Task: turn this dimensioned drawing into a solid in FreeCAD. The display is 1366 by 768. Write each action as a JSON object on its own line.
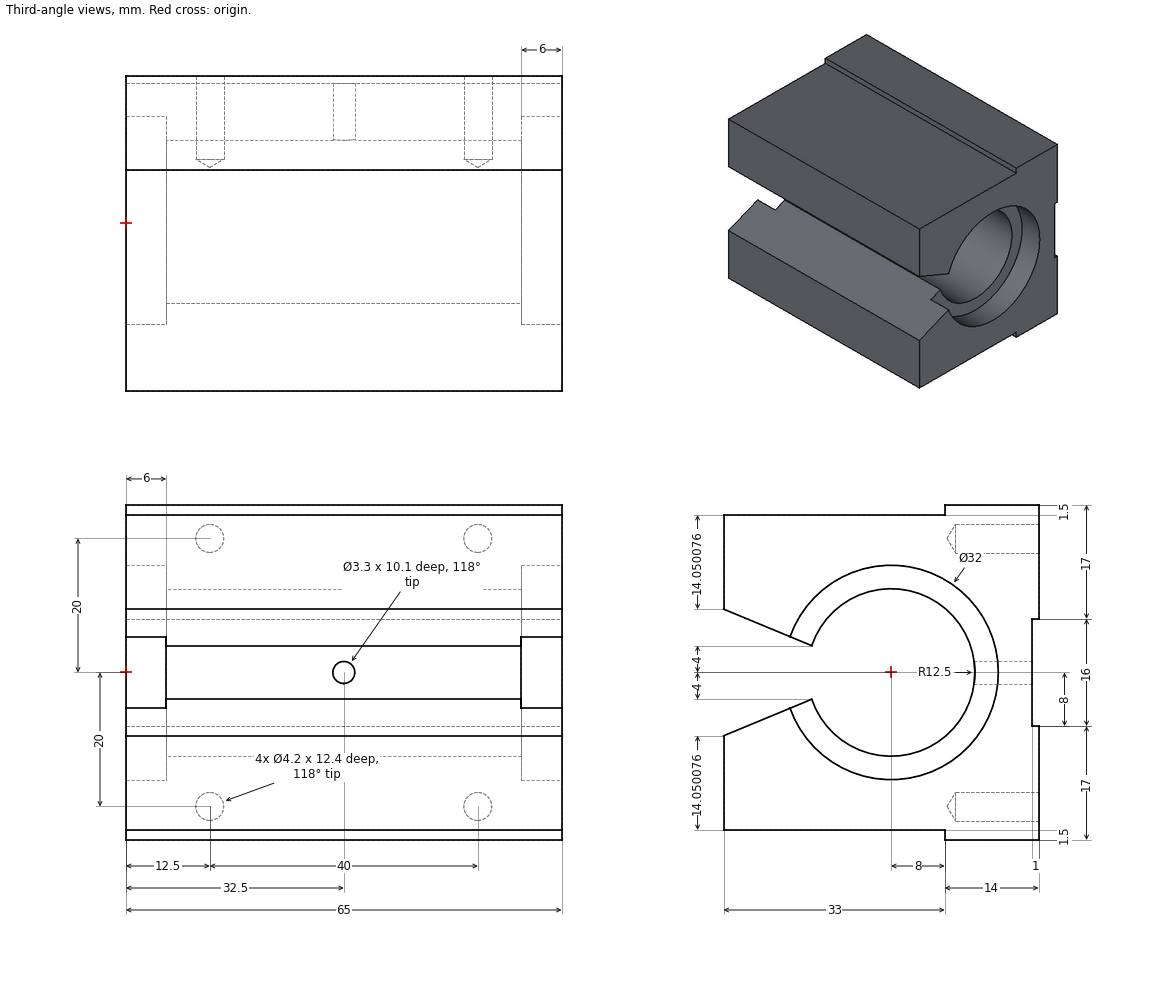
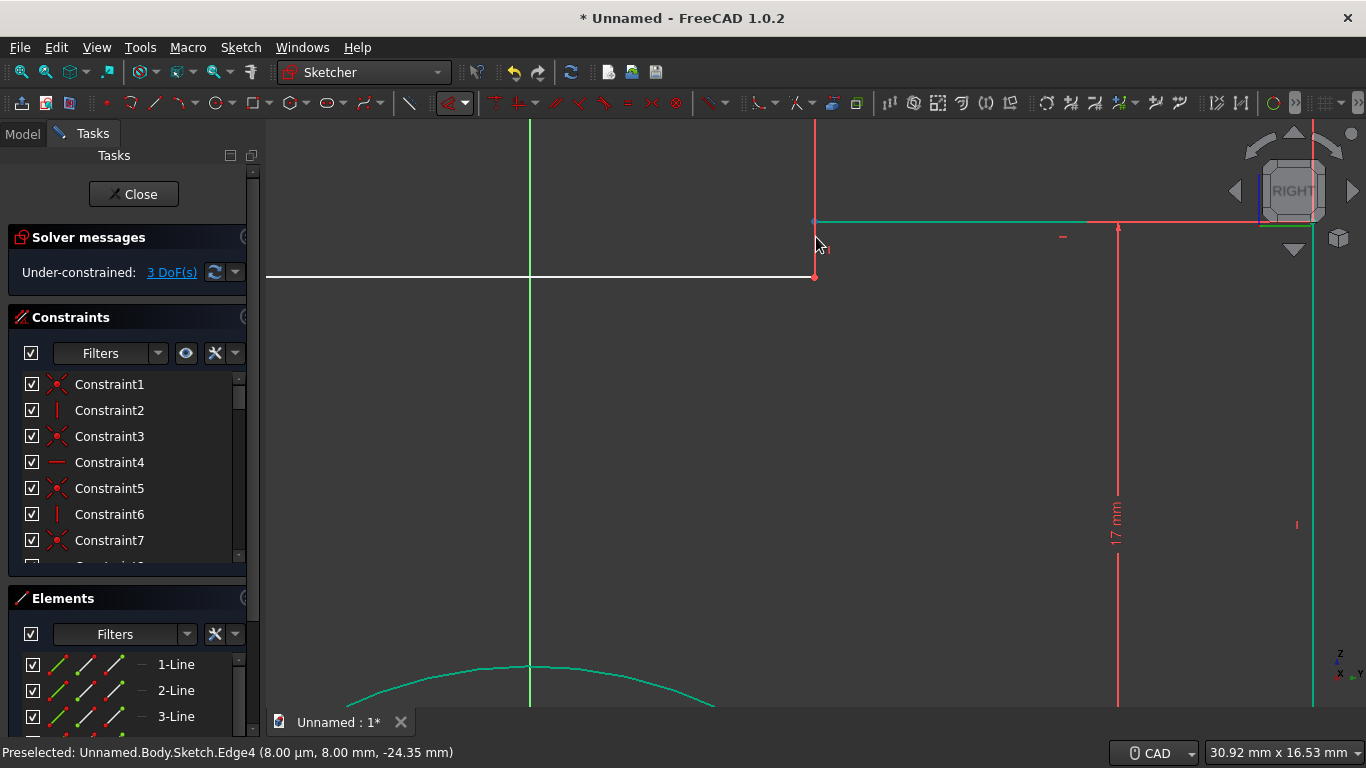
{"action": "left_click", "coordinate": [815, 238]}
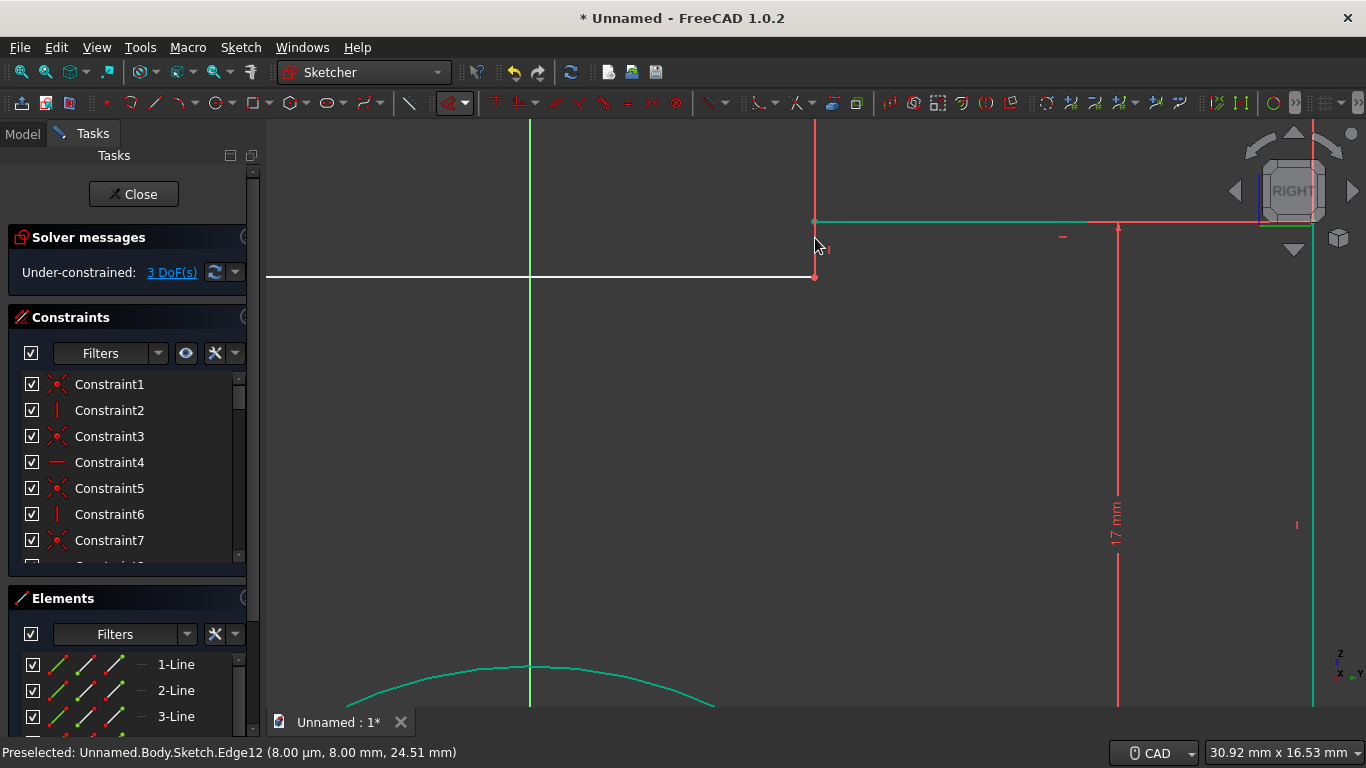
{"action": "key", "text": "i"}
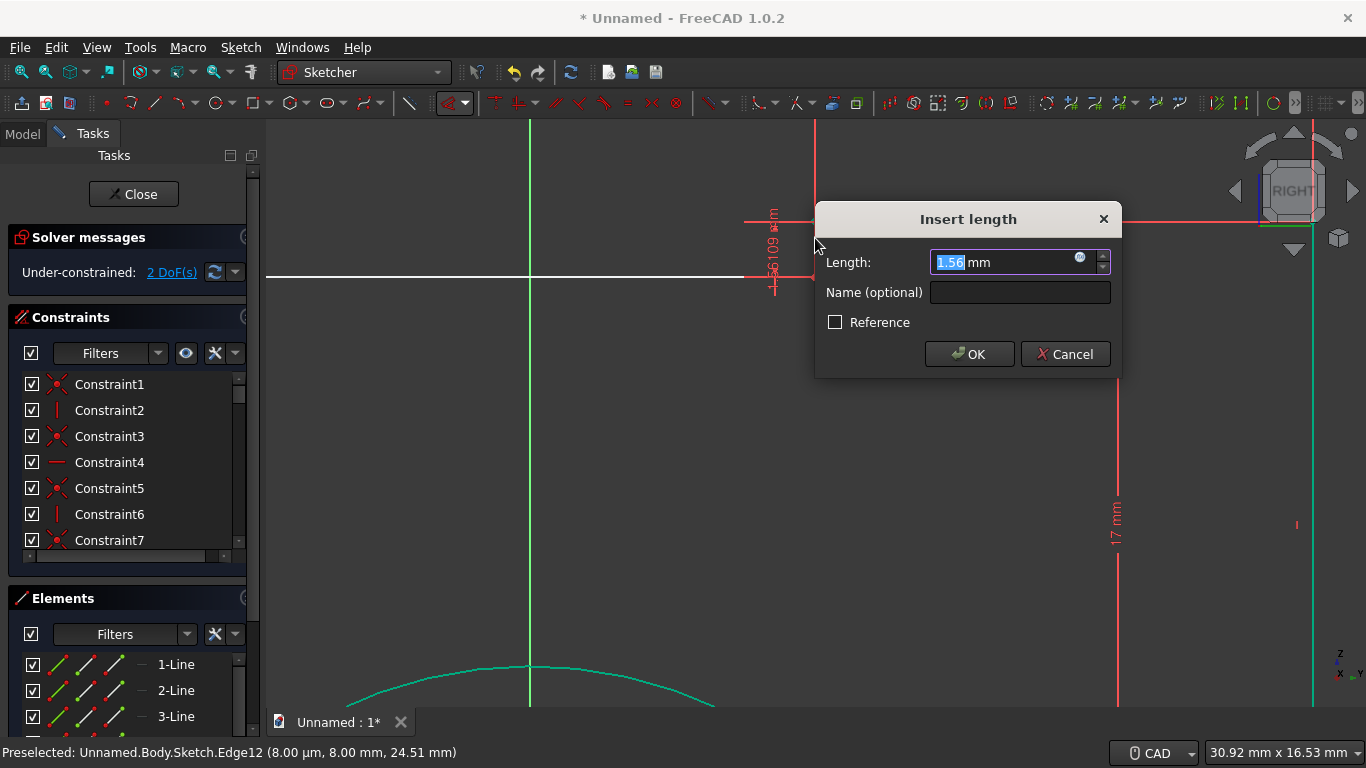
{"action": "type", "text": "1.5"}
{"action": "key", "text": "Return"}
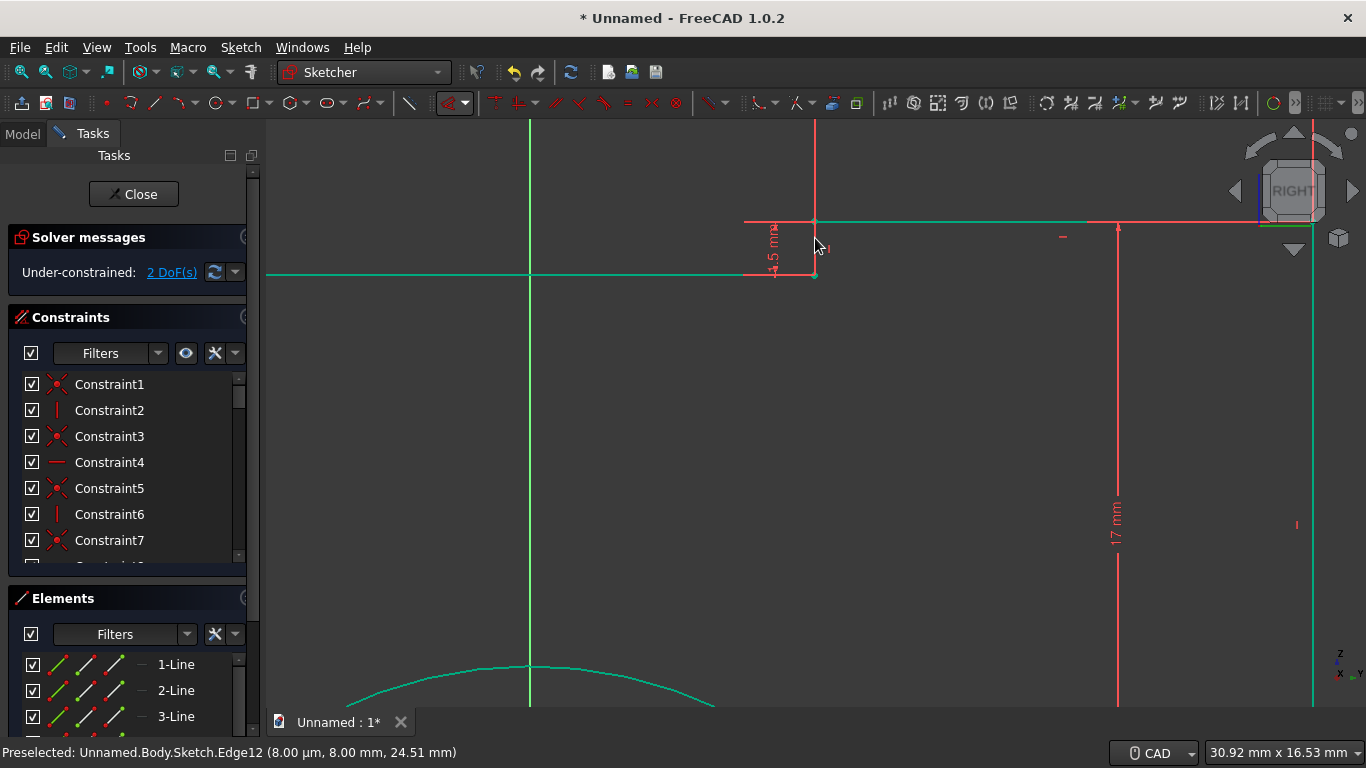
{"action": "scroll", "coordinate": [816, 236], "scroll_direction": "down", "scroll_amount": 8}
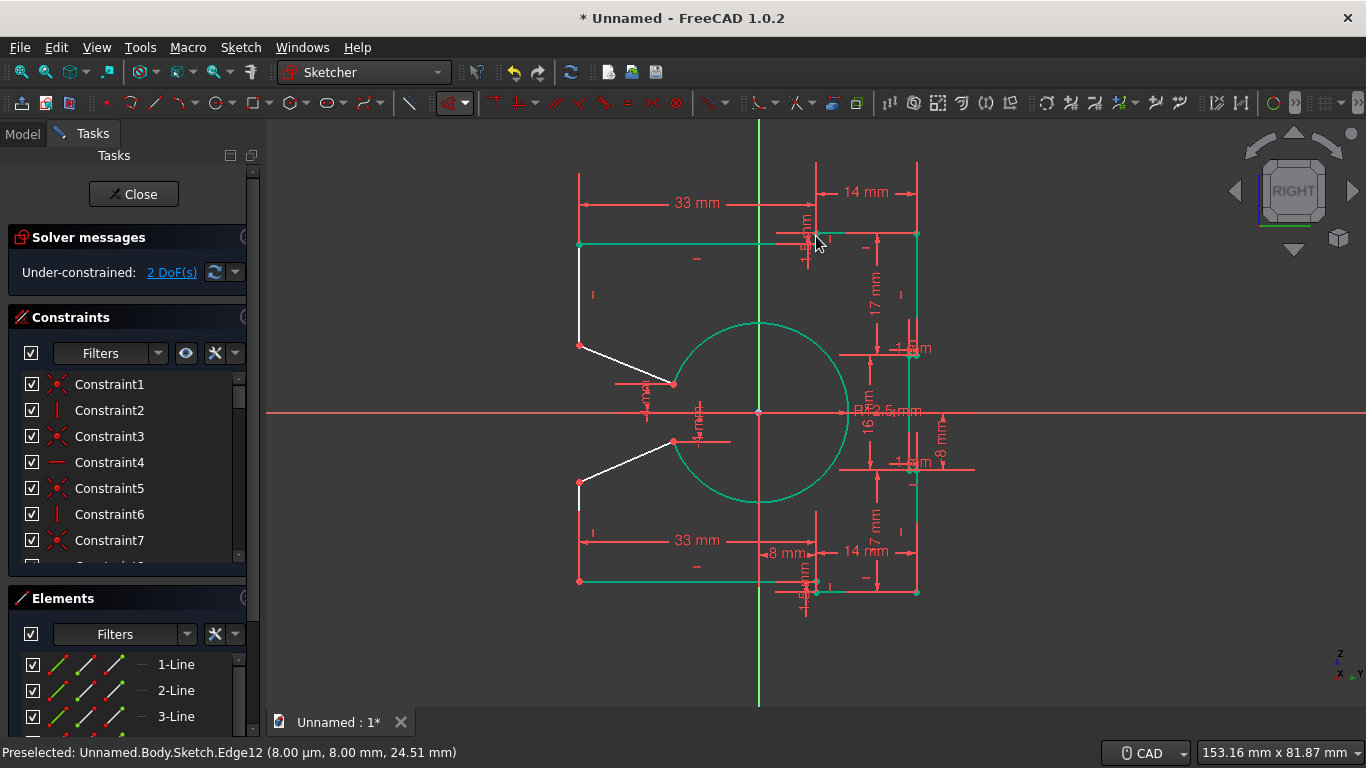
{"action": "left_click", "coordinate": [579, 512]}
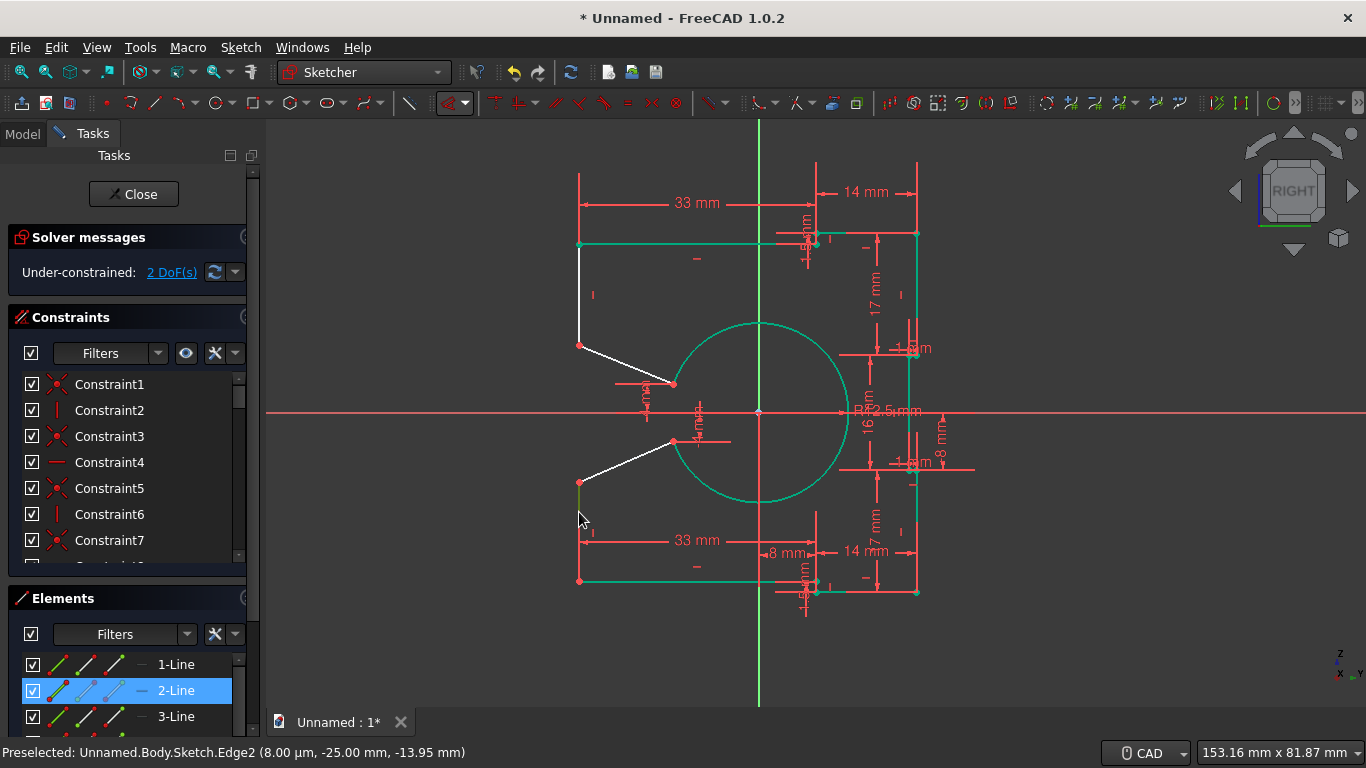
{"action": "key", "text": "i"}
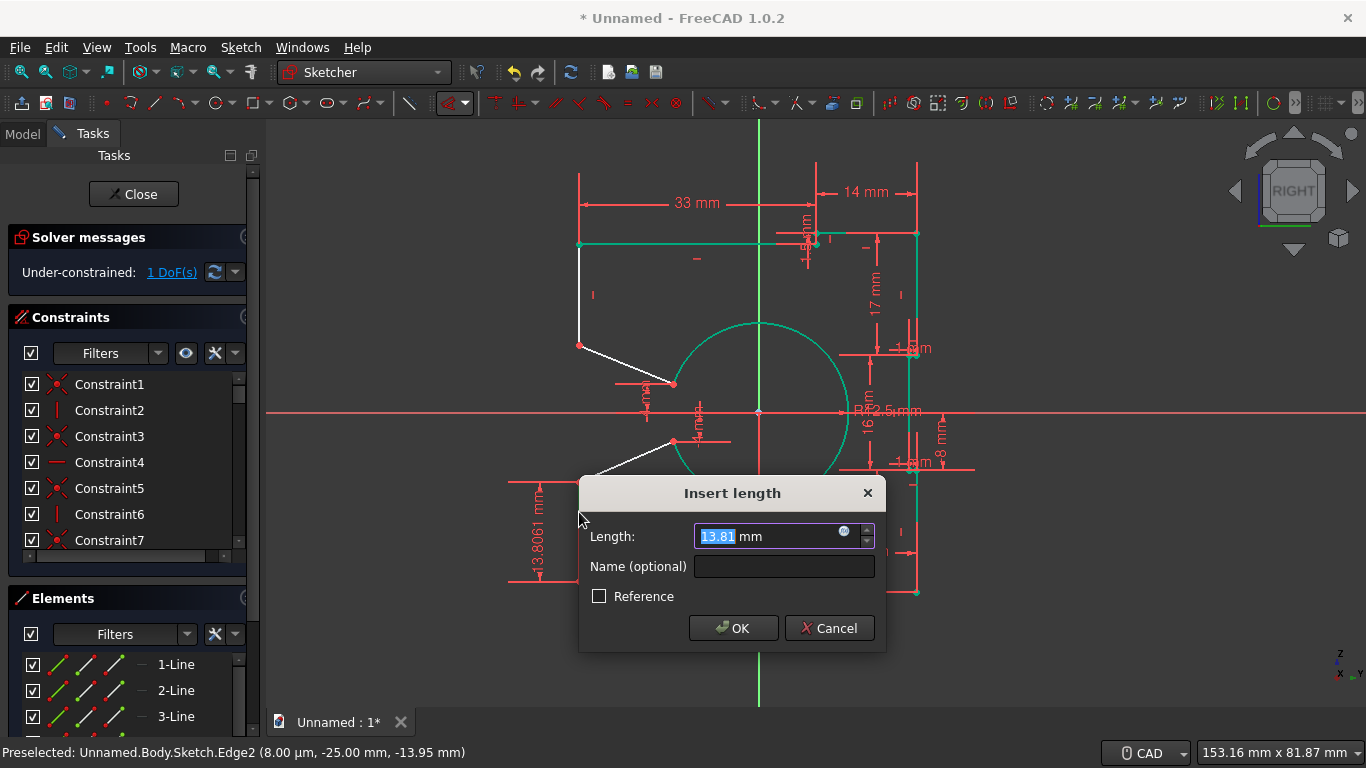
{"action": "type", "text": "14.050076"}
{"action": "key", "text": "Return"}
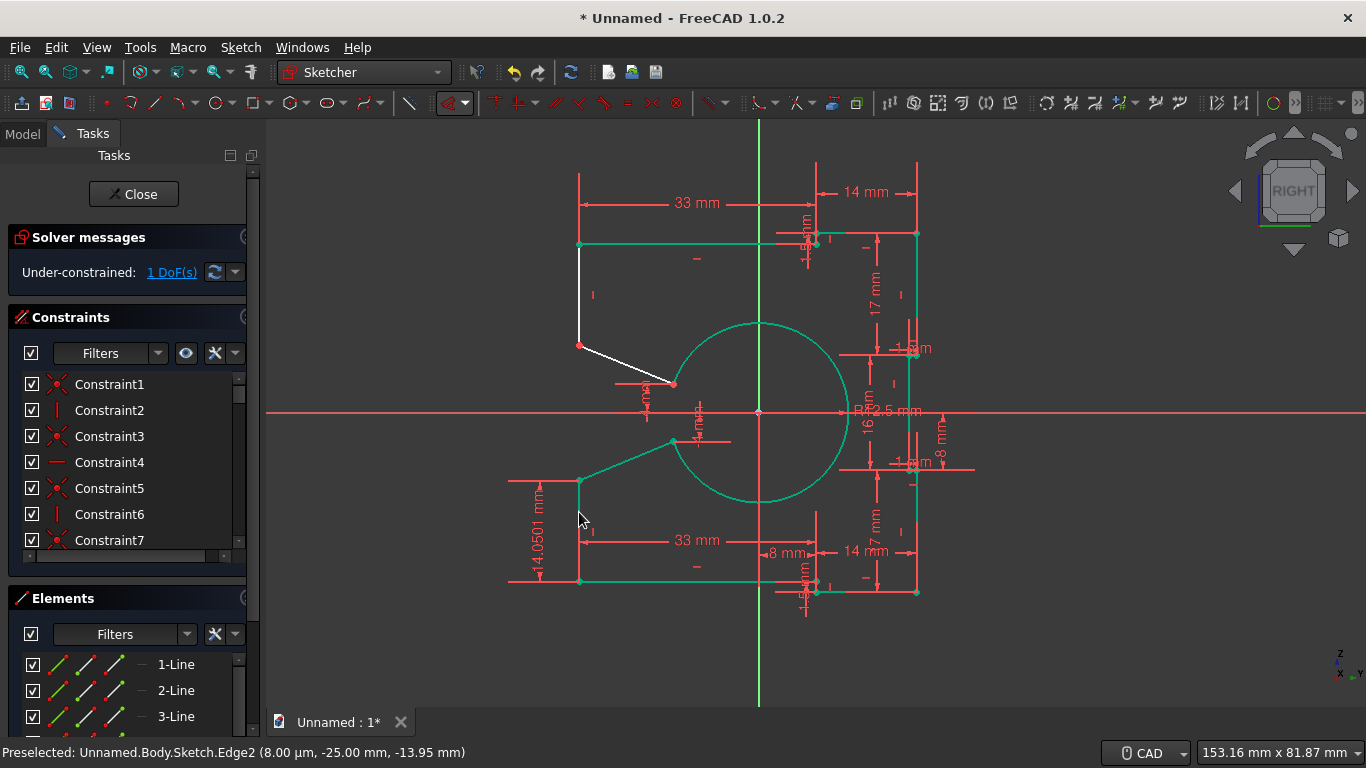
{"action": "left_click", "coordinate": [579, 275]}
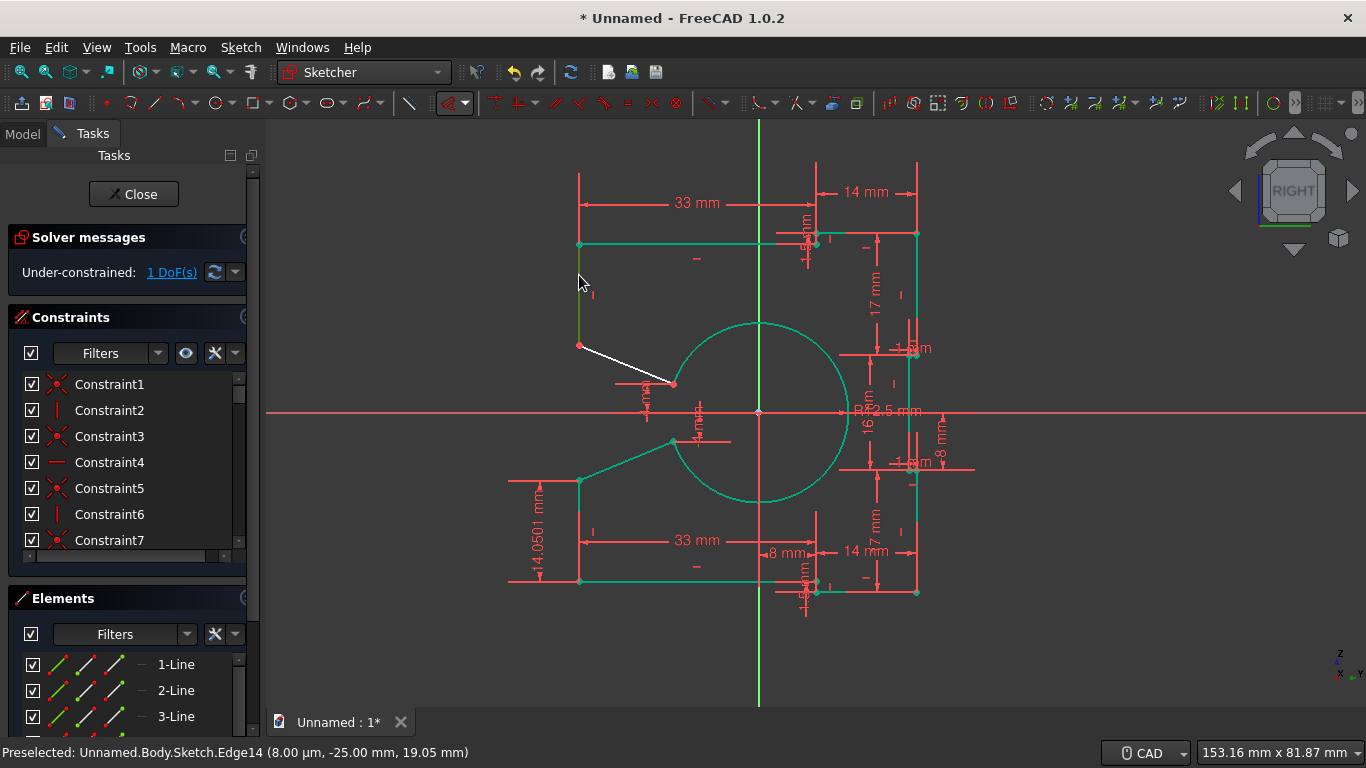
{"action": "left_click", "coordinate": [468, 104]}